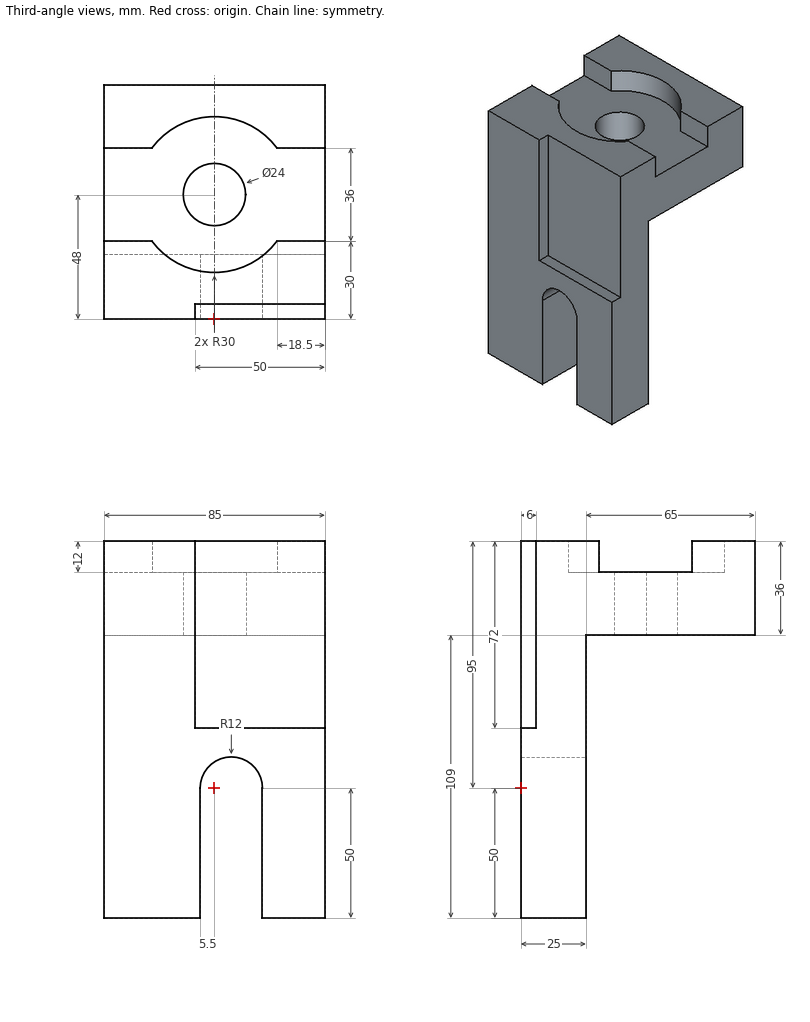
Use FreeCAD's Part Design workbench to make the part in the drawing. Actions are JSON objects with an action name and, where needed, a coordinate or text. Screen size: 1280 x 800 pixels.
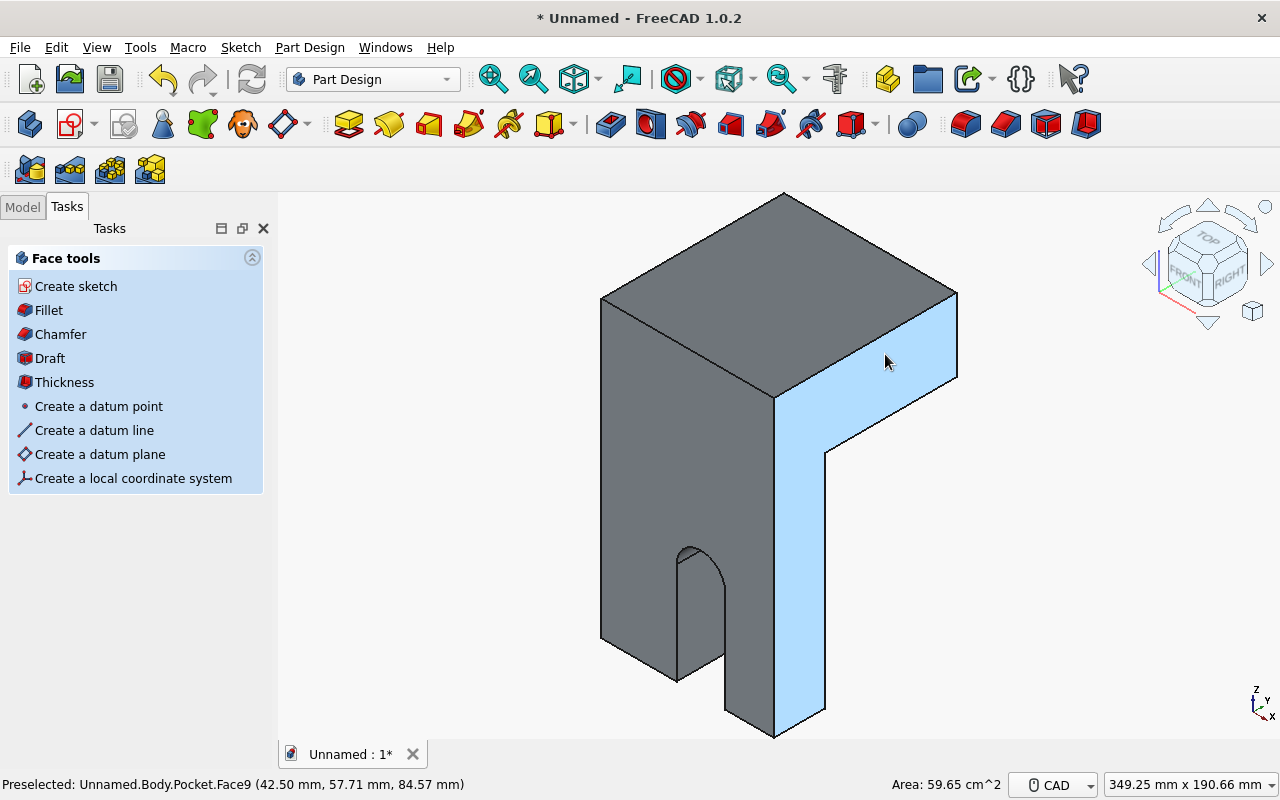
{"action": "left_click", "coordinate": [70, 124]}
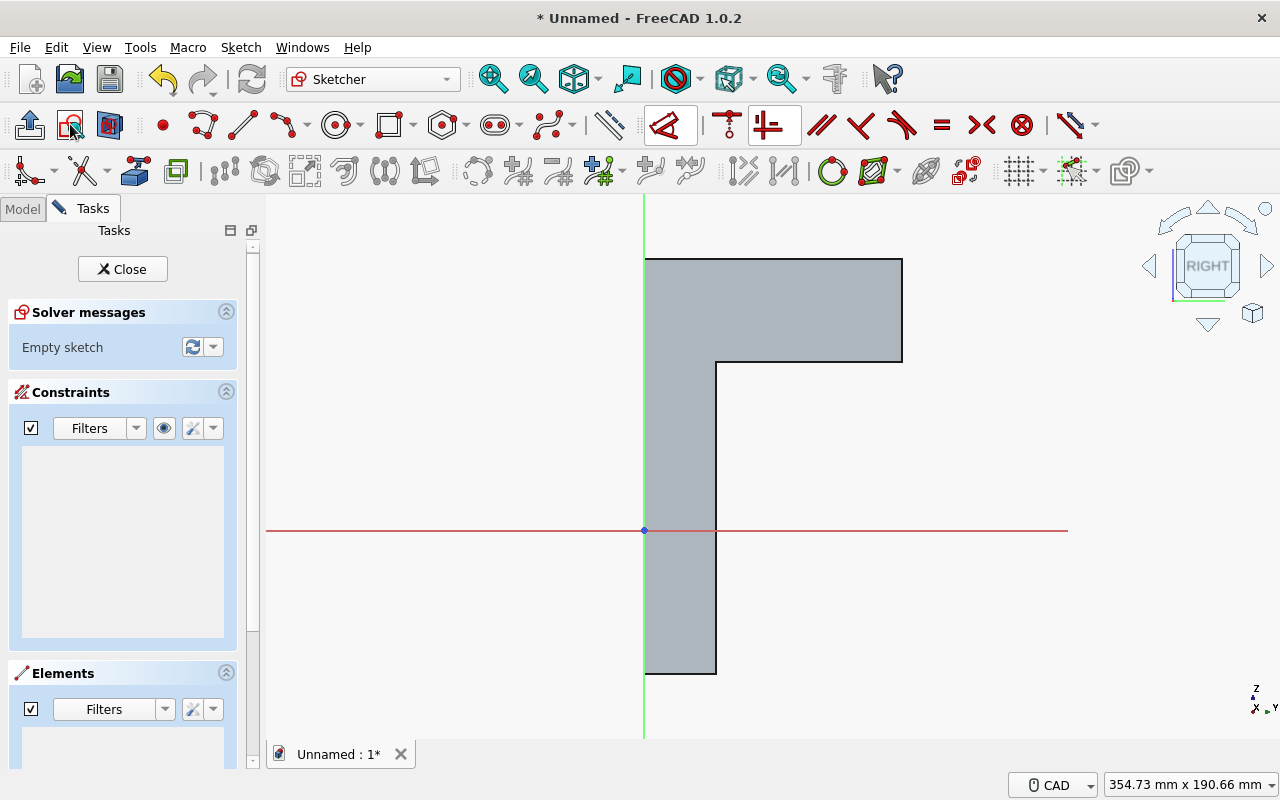
{"action": "left_click", "coordinate": [390, 126]}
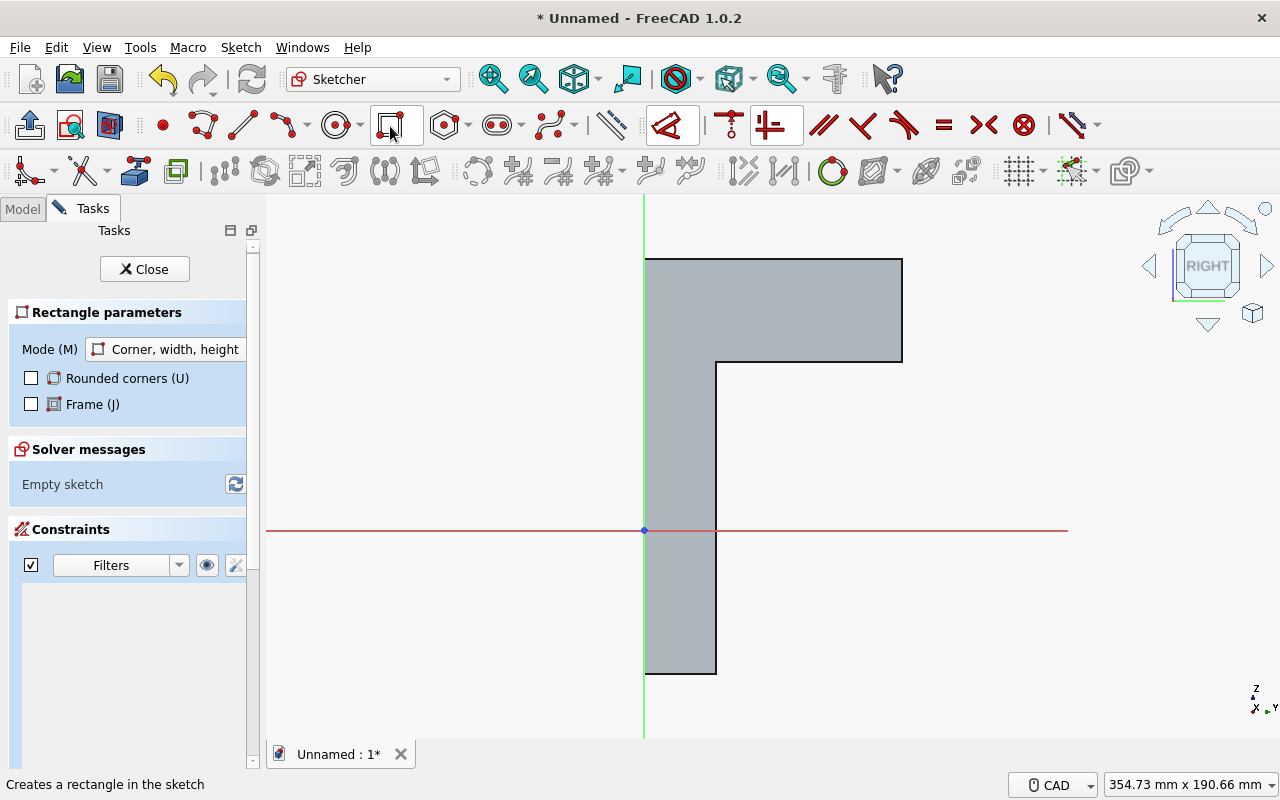
{"action": "left_click", "coordinate": [644, 259]}
{"action": "left_click", "coordinate": [662, 465]}
{"action": "key", "text": "Escape"}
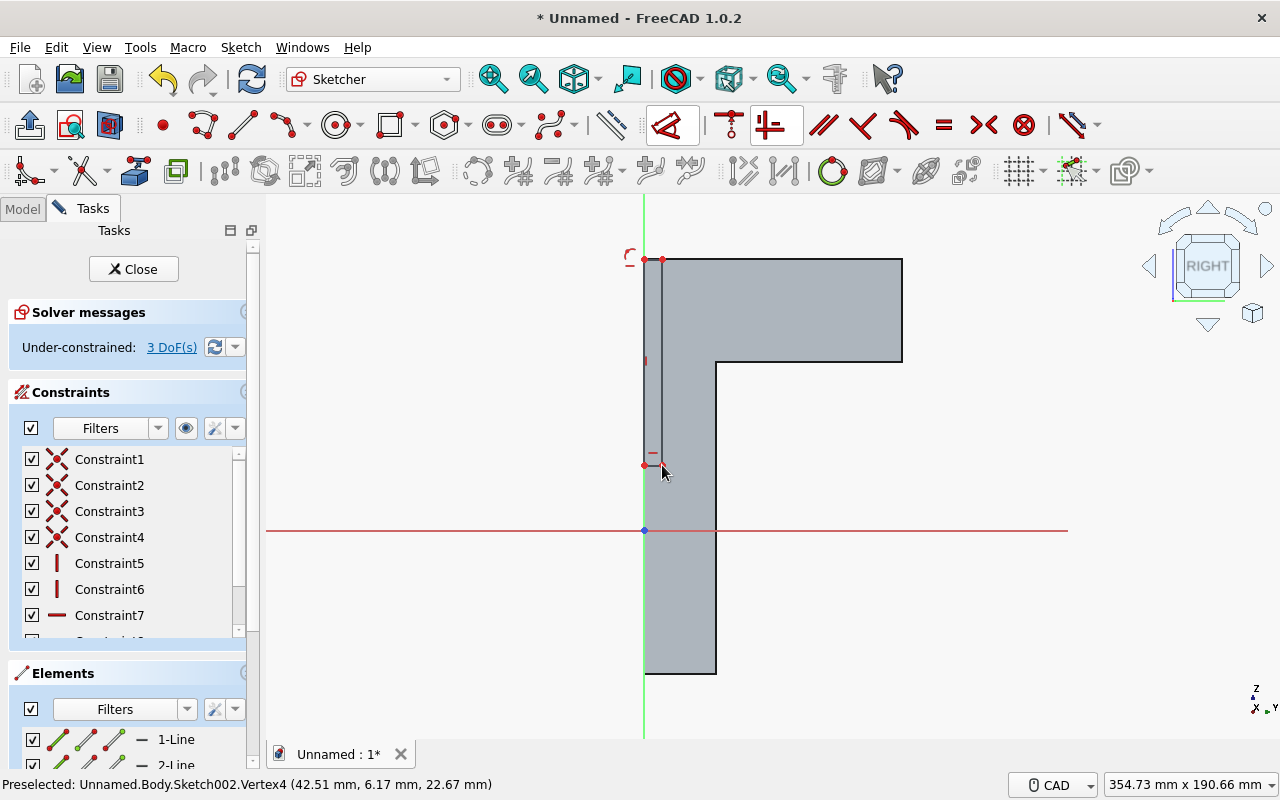
{"action": "scroll", "coordinate": [653, 466], "scroll_direction": "up", "scroll_amount": 5}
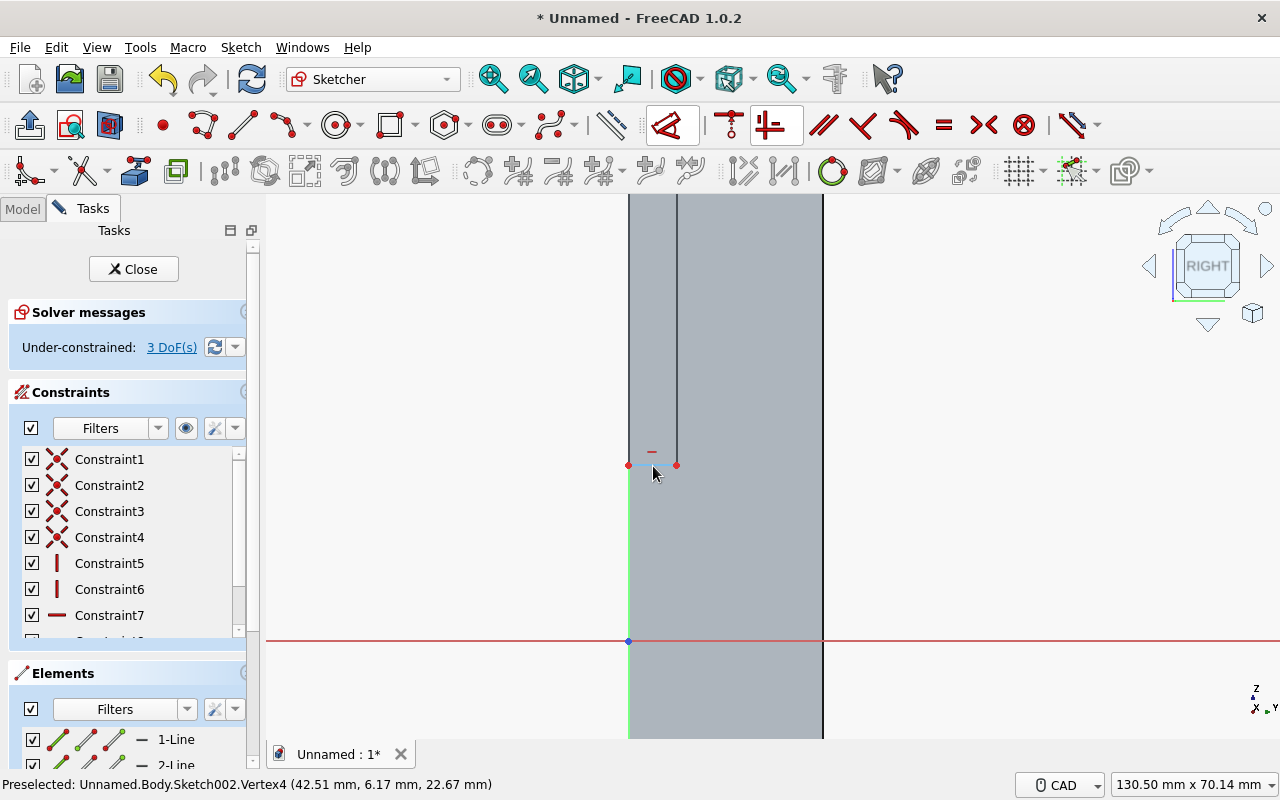
{"action": "left_click", "coordinate": [653, 465]}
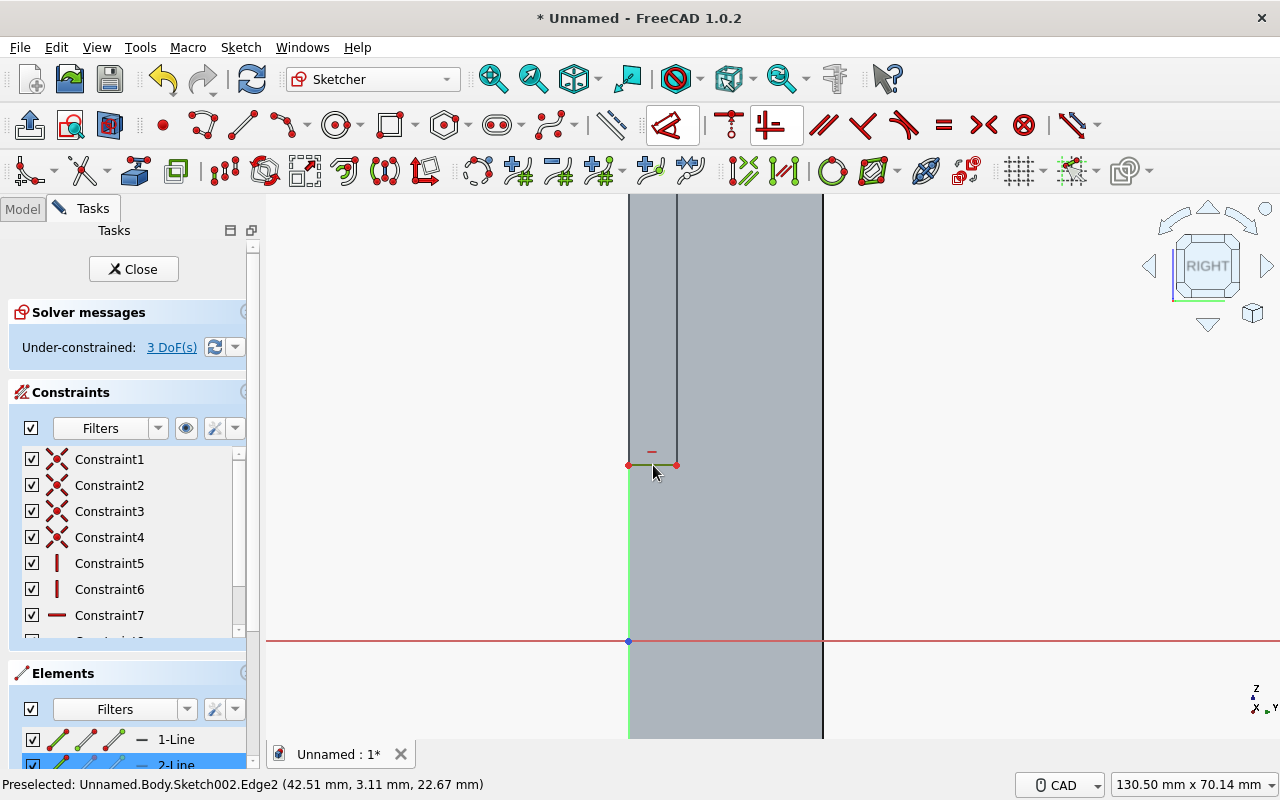
{"action": "key", "text": "l"}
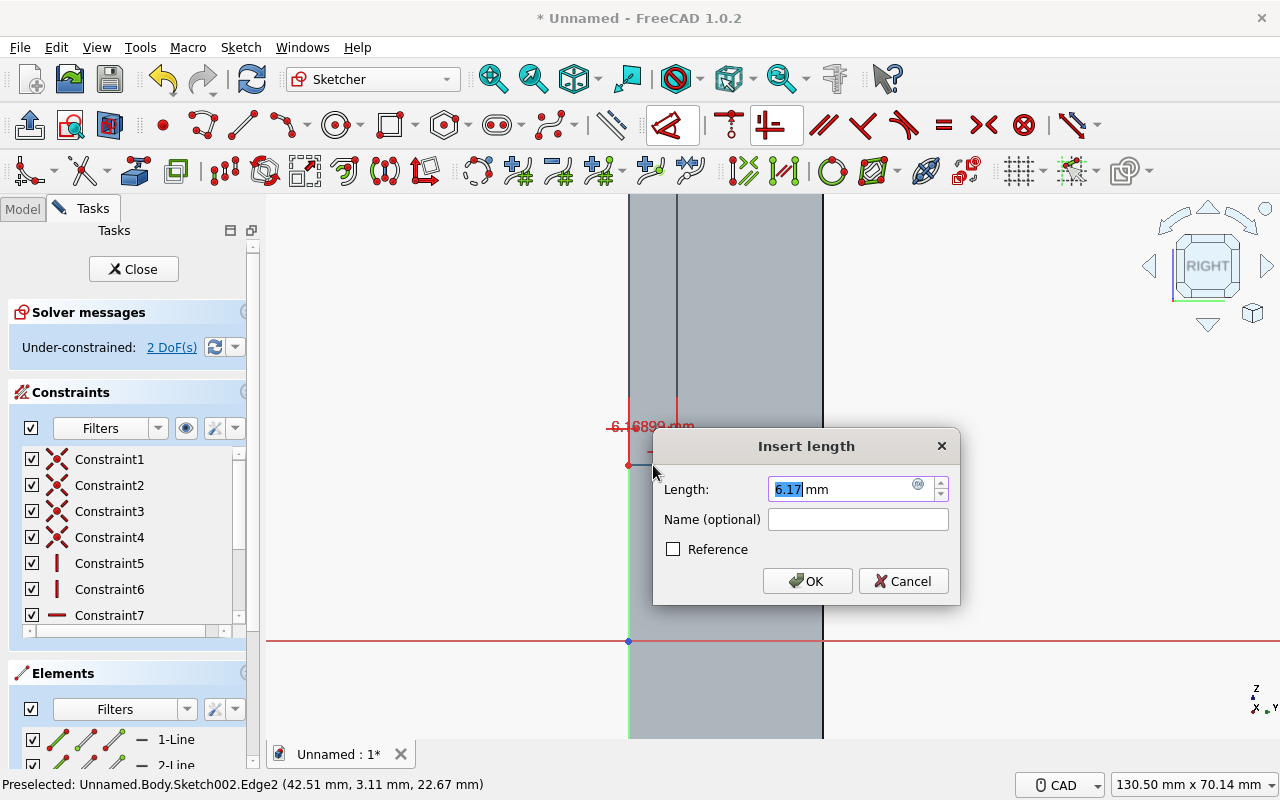
{"action": "type", "text": "6"}
{"action": "key", "text": "Return"}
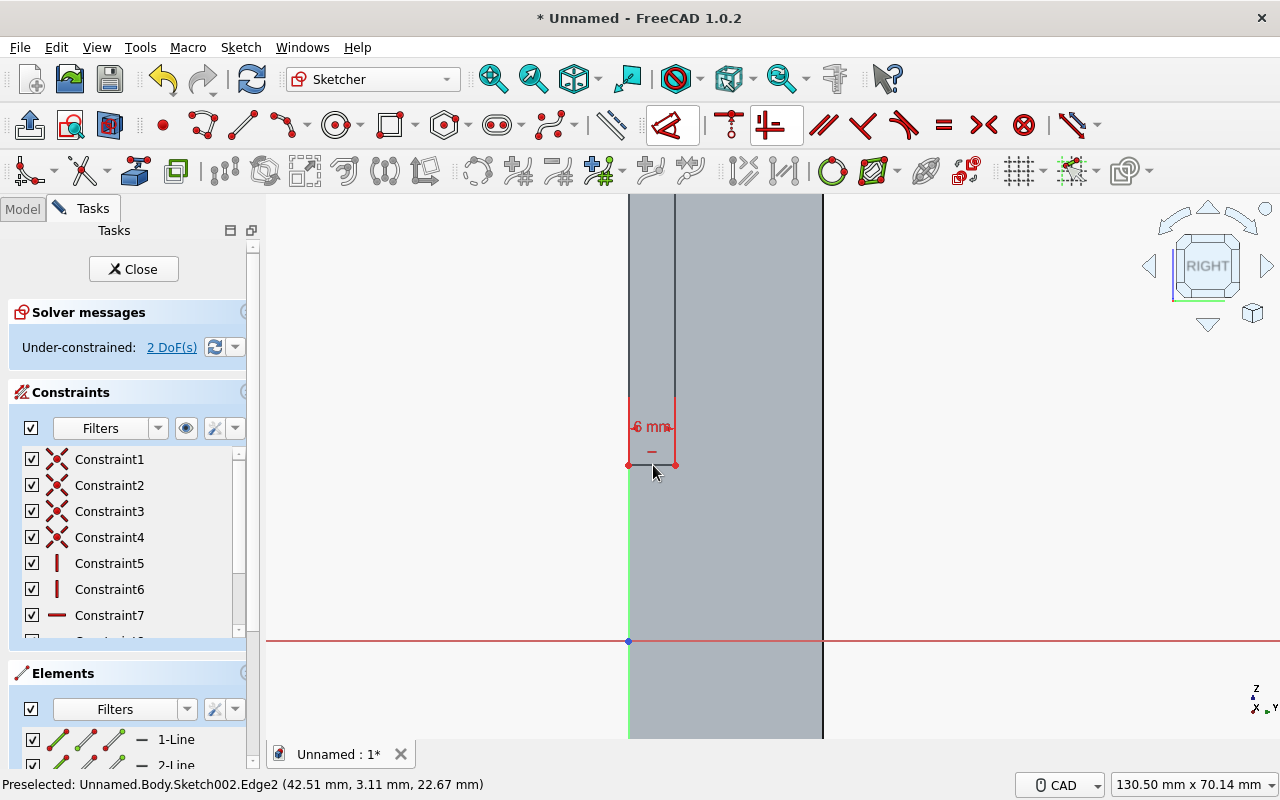
{"action": "left_click", "coordinate": [629, 297]}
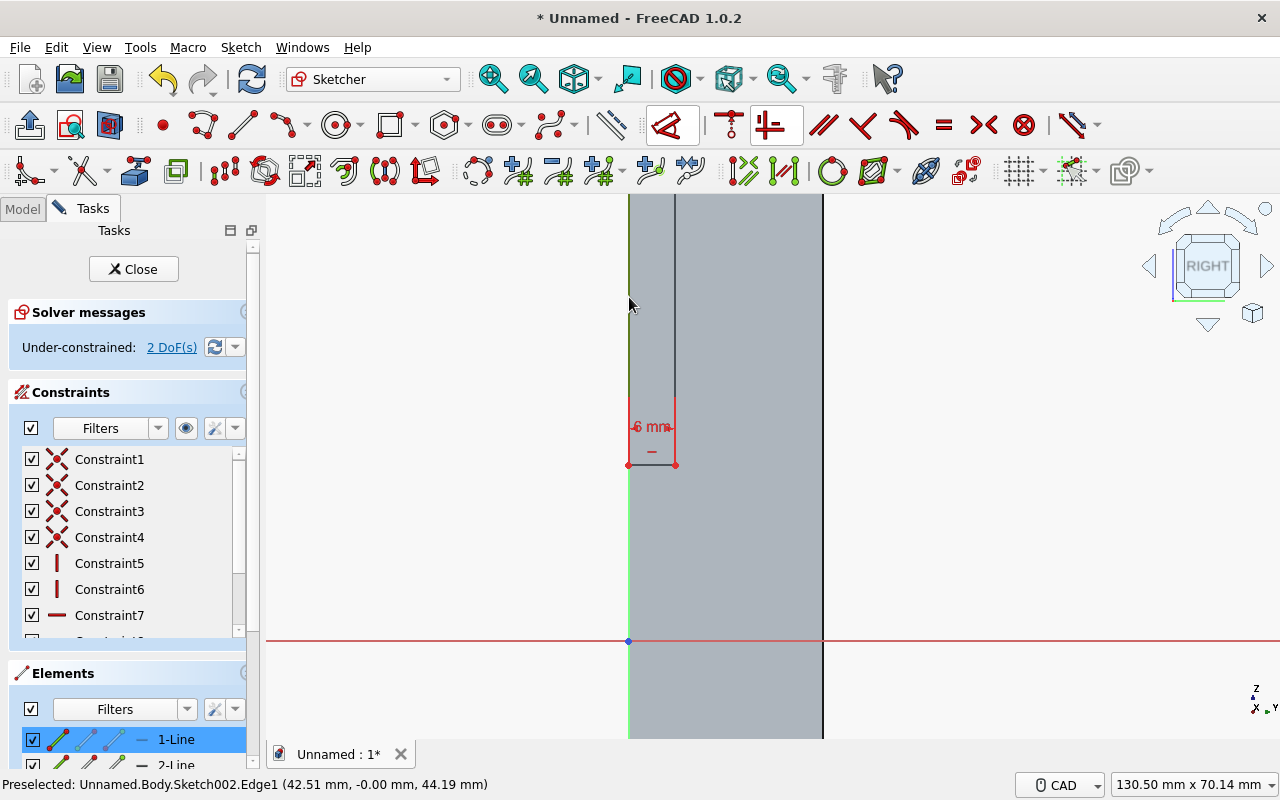
{"action": "left_click", "coordinate": [694, 126]}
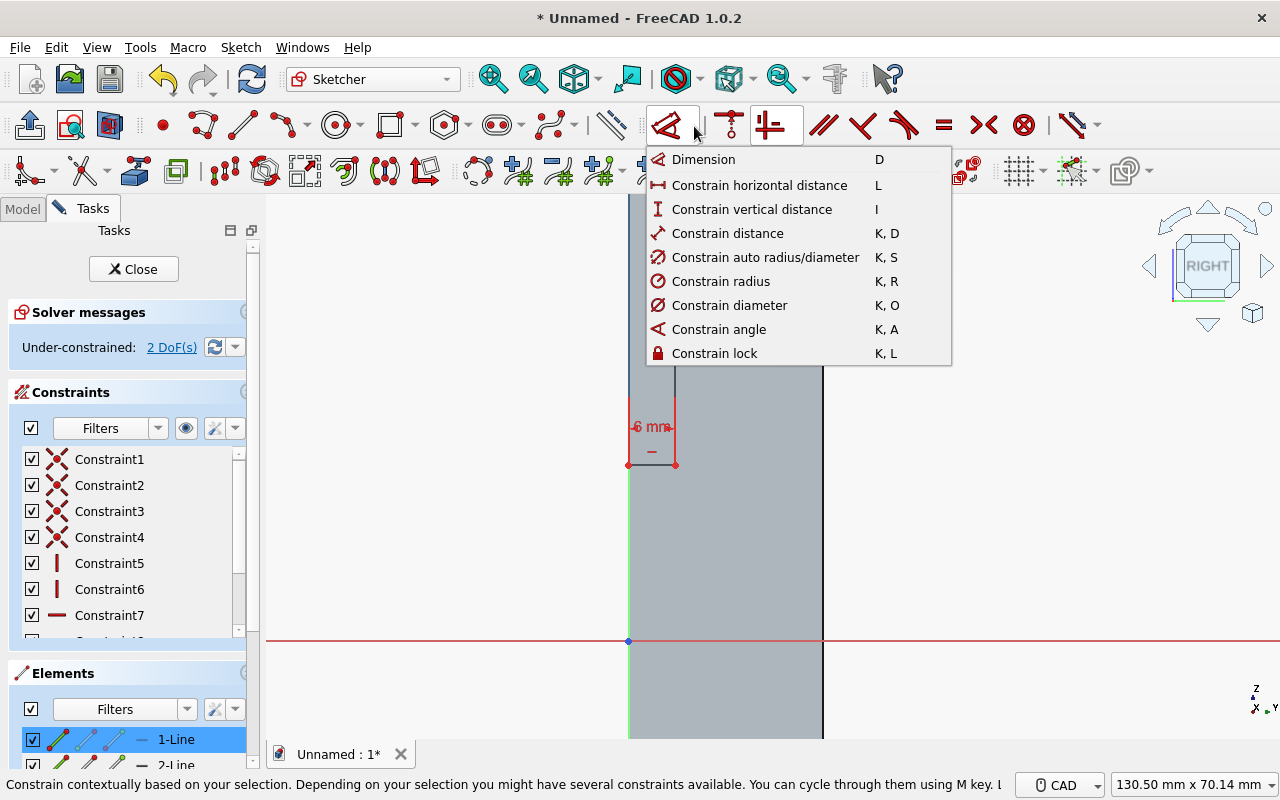
{"action": "left_click", "coordinate": [799, 209]}